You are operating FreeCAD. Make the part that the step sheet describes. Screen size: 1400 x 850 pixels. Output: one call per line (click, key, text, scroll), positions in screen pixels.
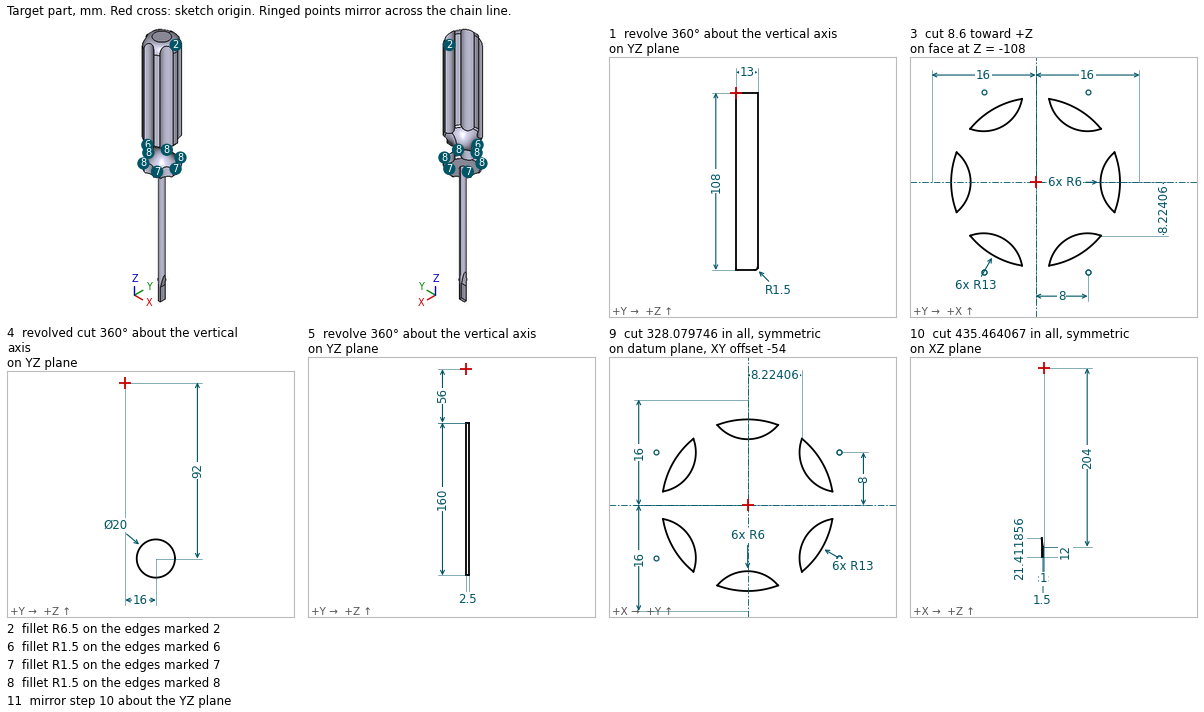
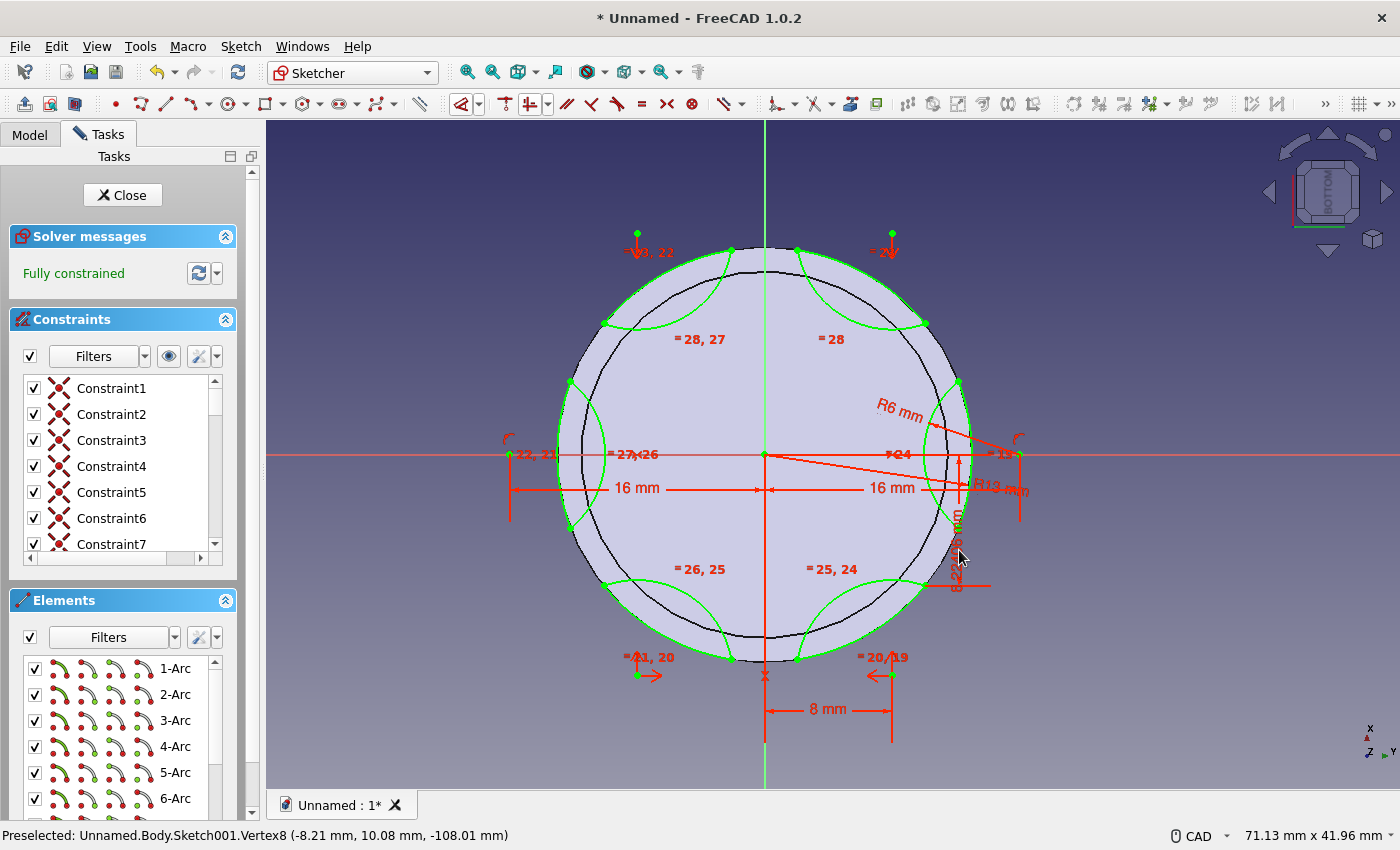
click(123, 195)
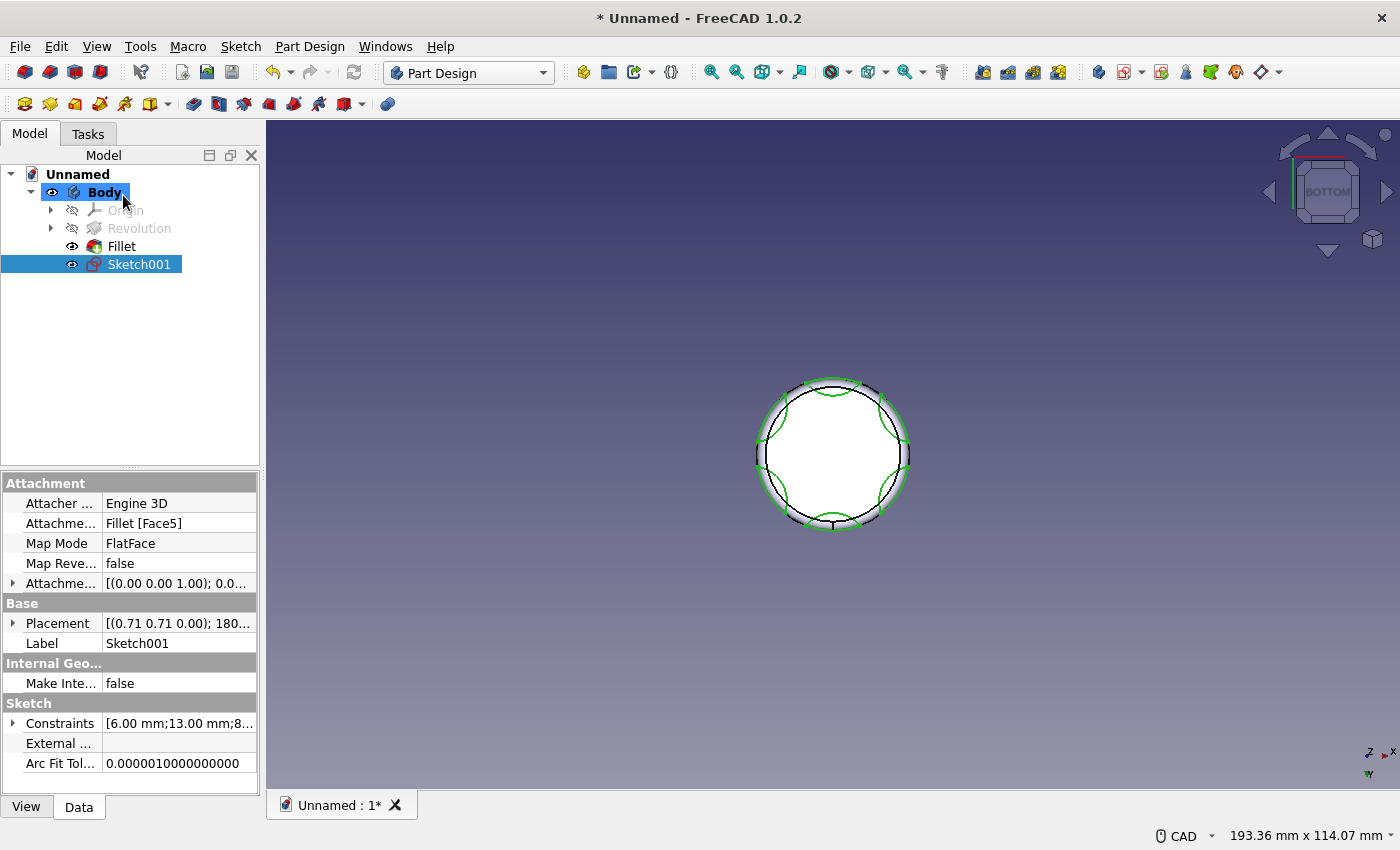
click(194, 104)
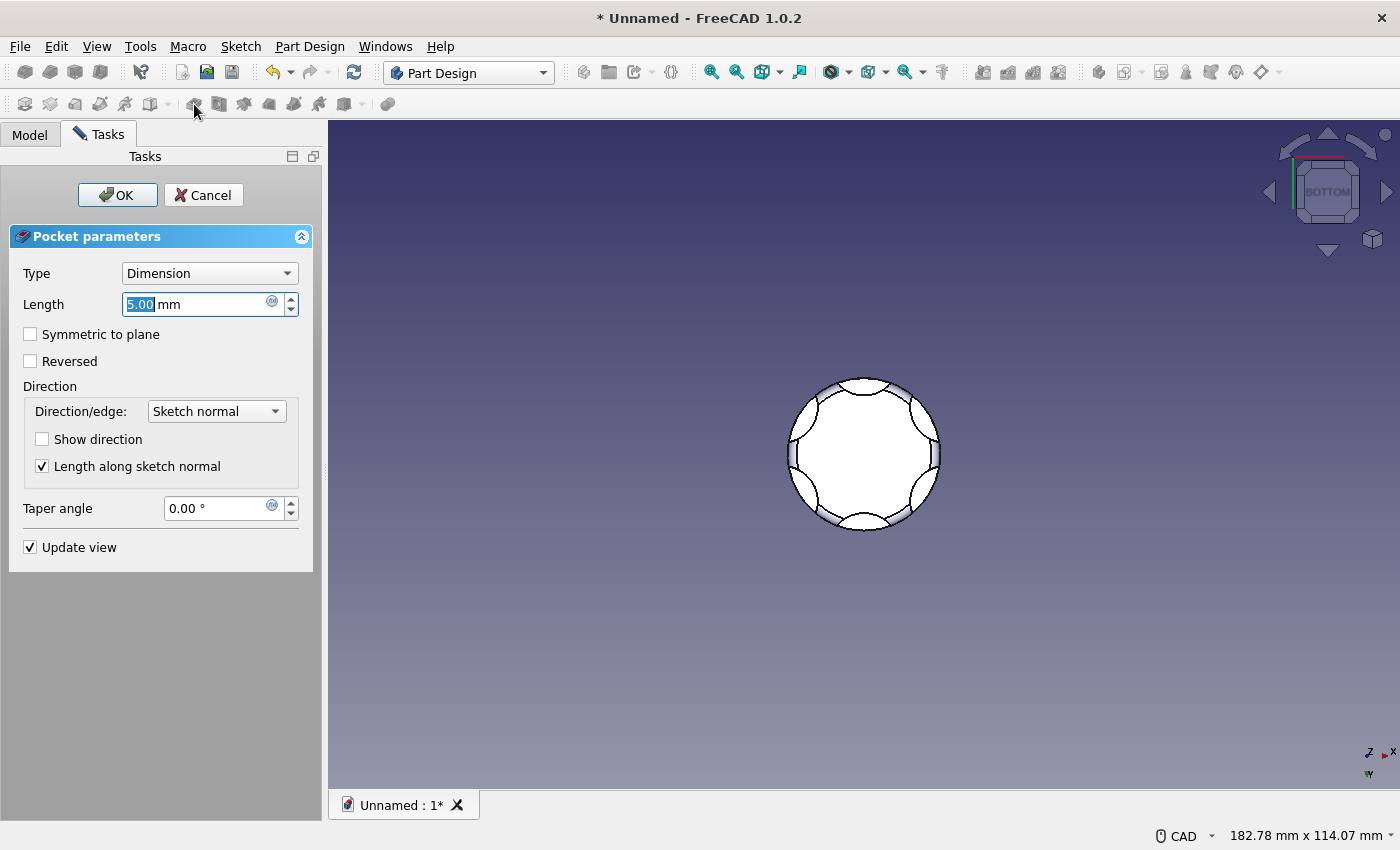
text(8.6)
key(Tab)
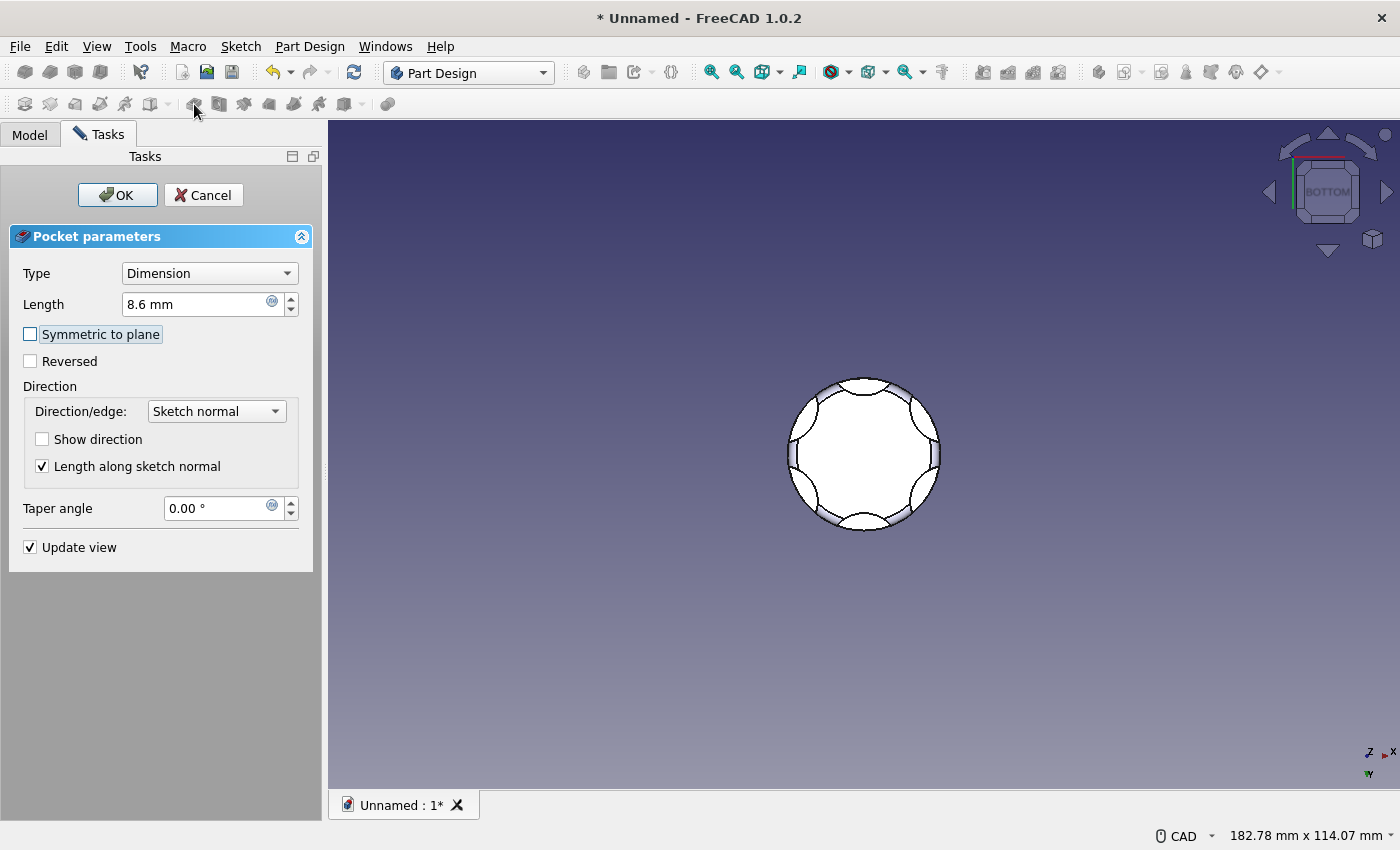
click(118, 195)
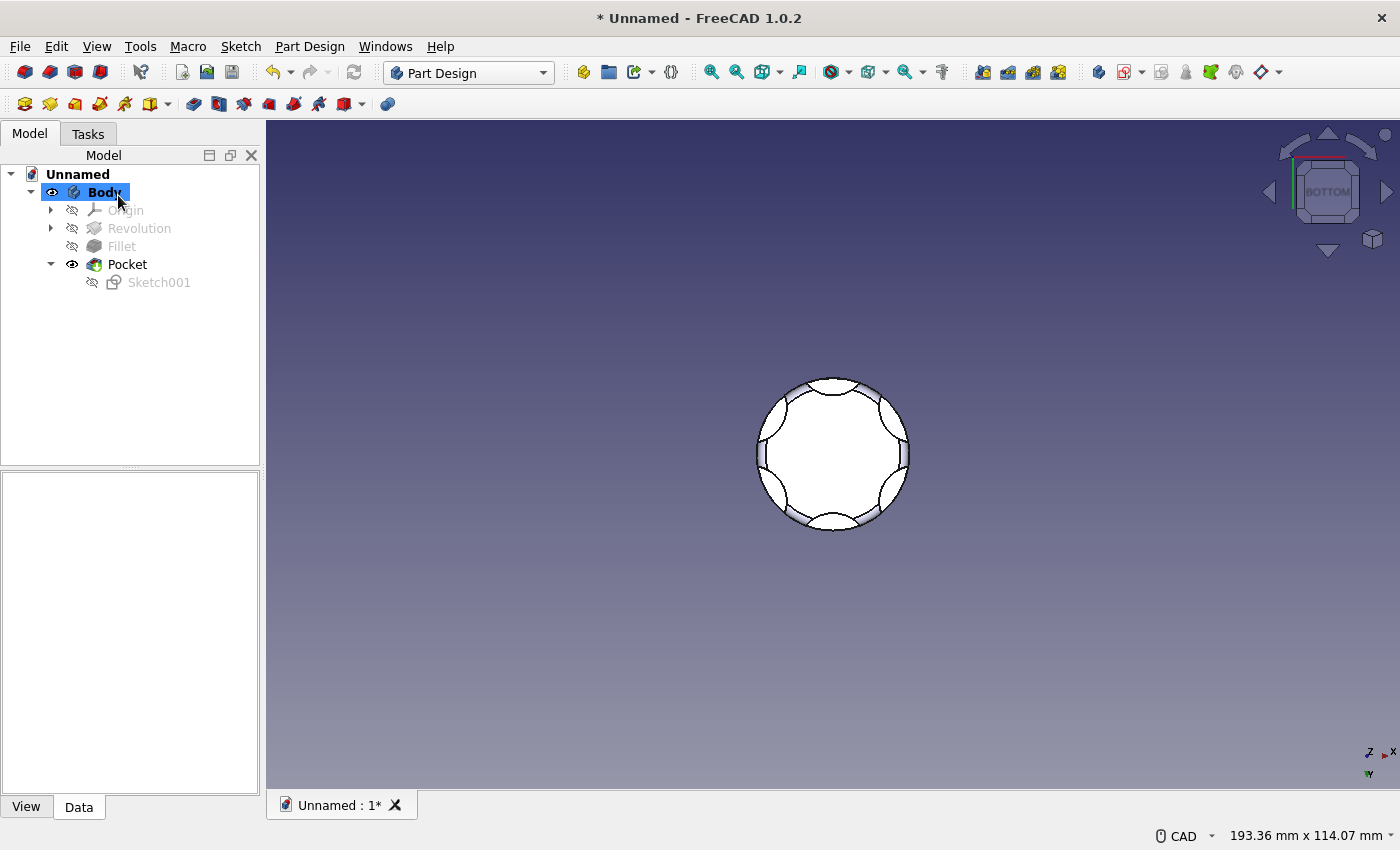
key(v)
key(f)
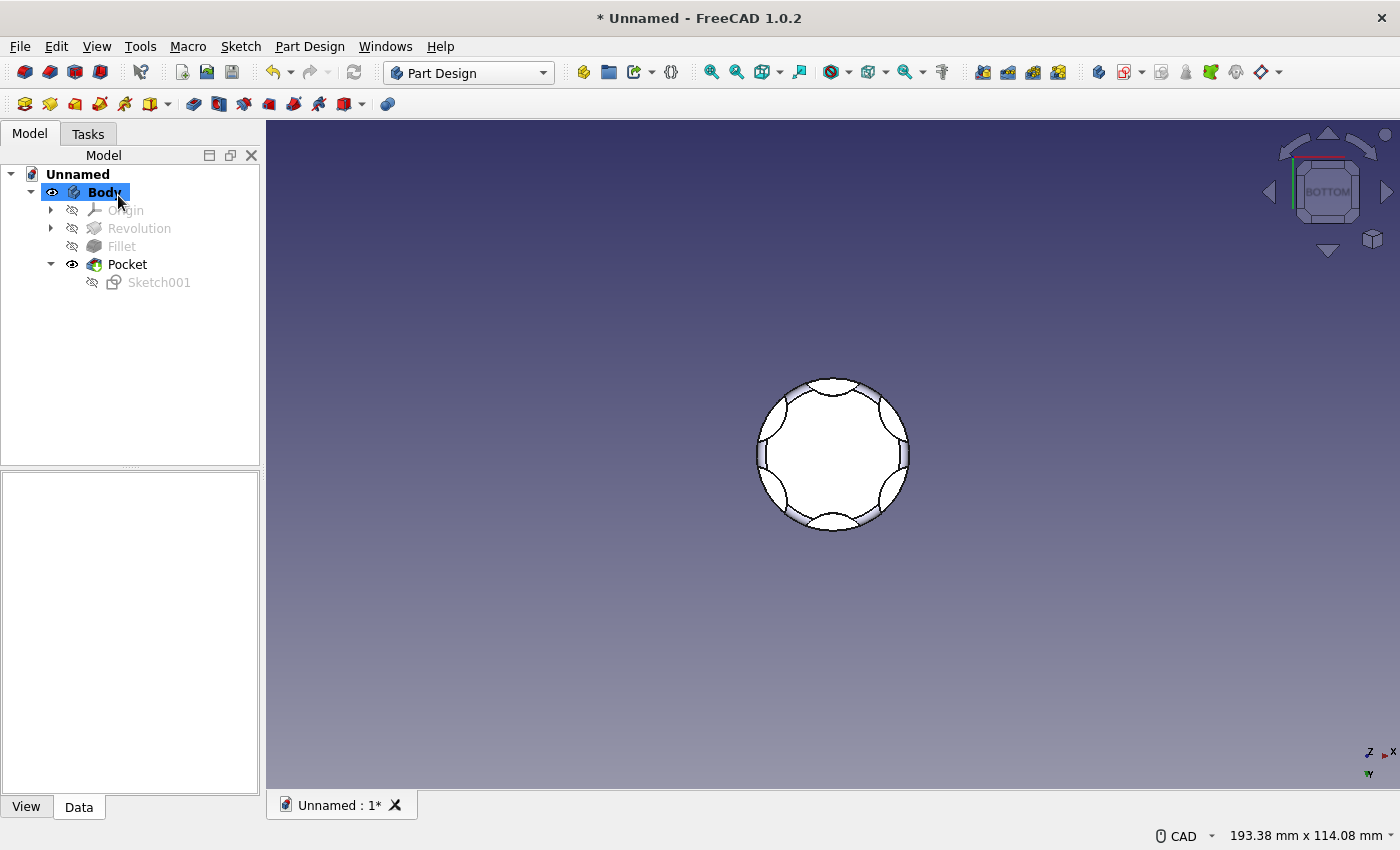
click(1124, 72)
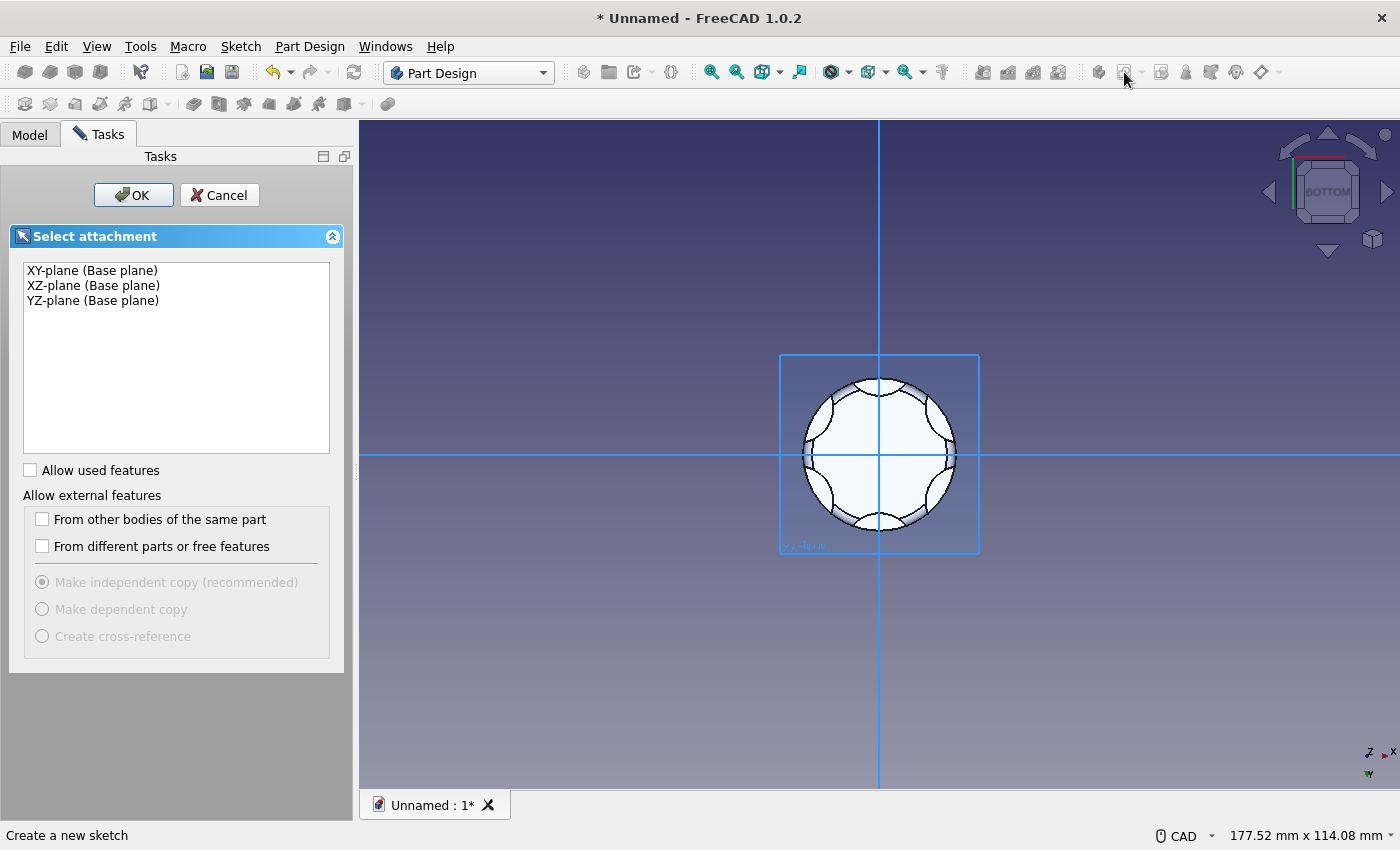
click(84, 300)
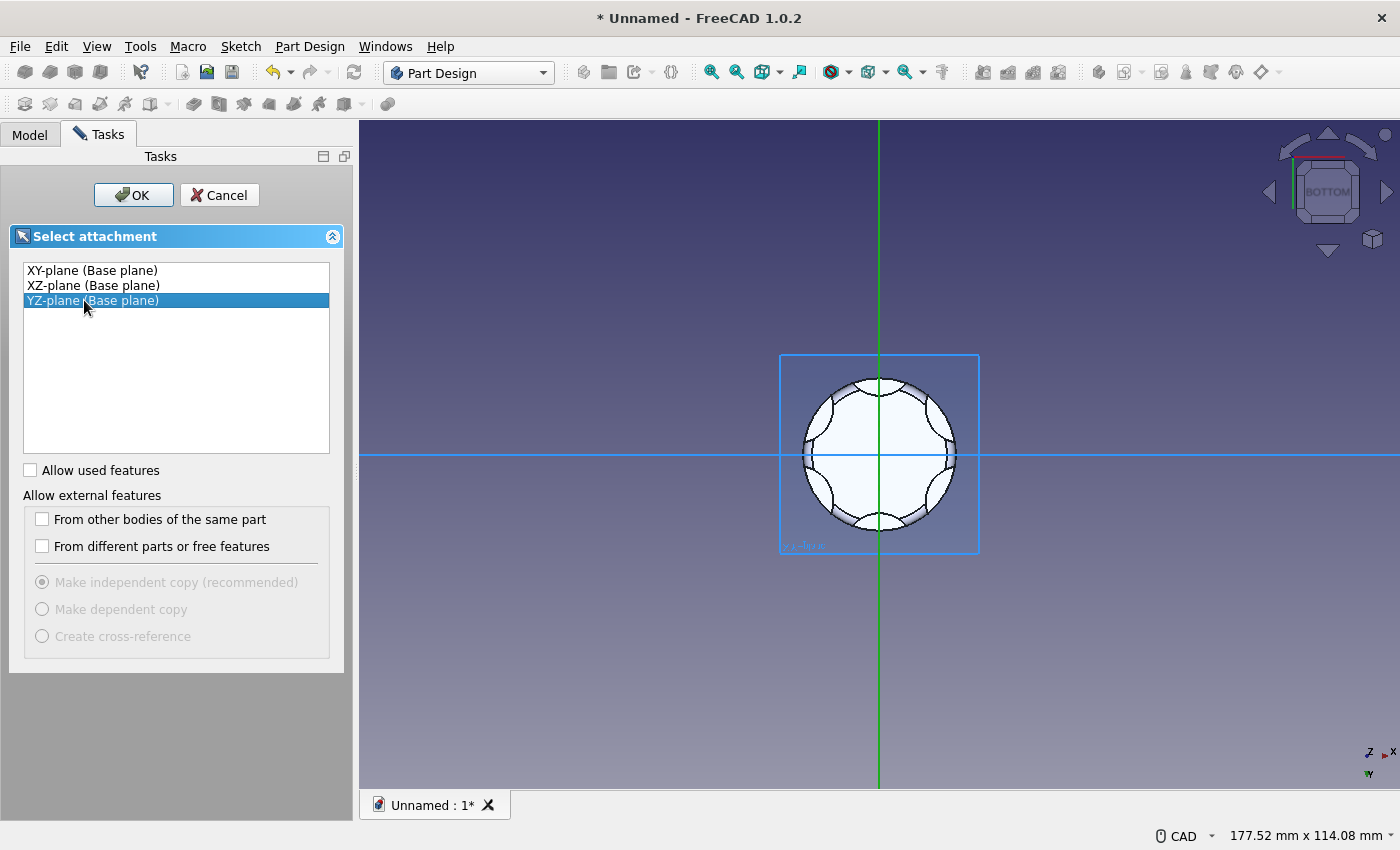
click(134, 195)